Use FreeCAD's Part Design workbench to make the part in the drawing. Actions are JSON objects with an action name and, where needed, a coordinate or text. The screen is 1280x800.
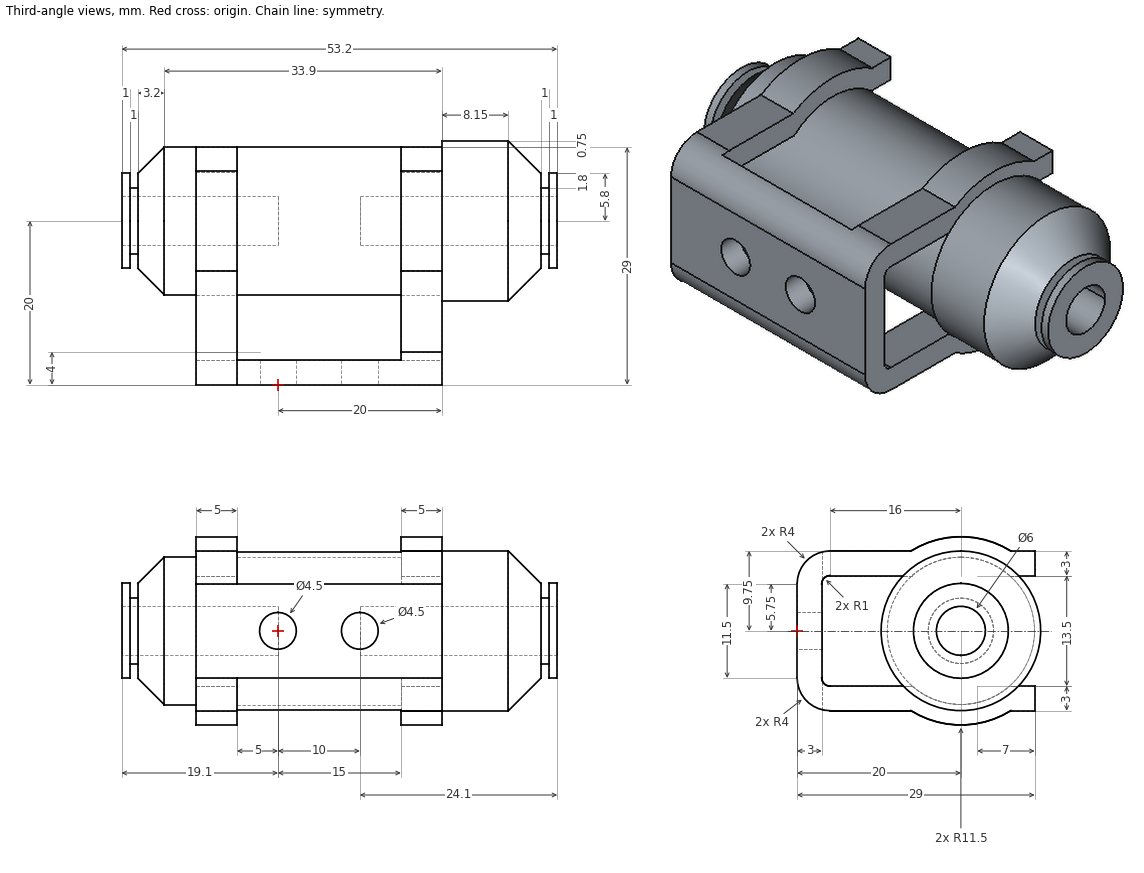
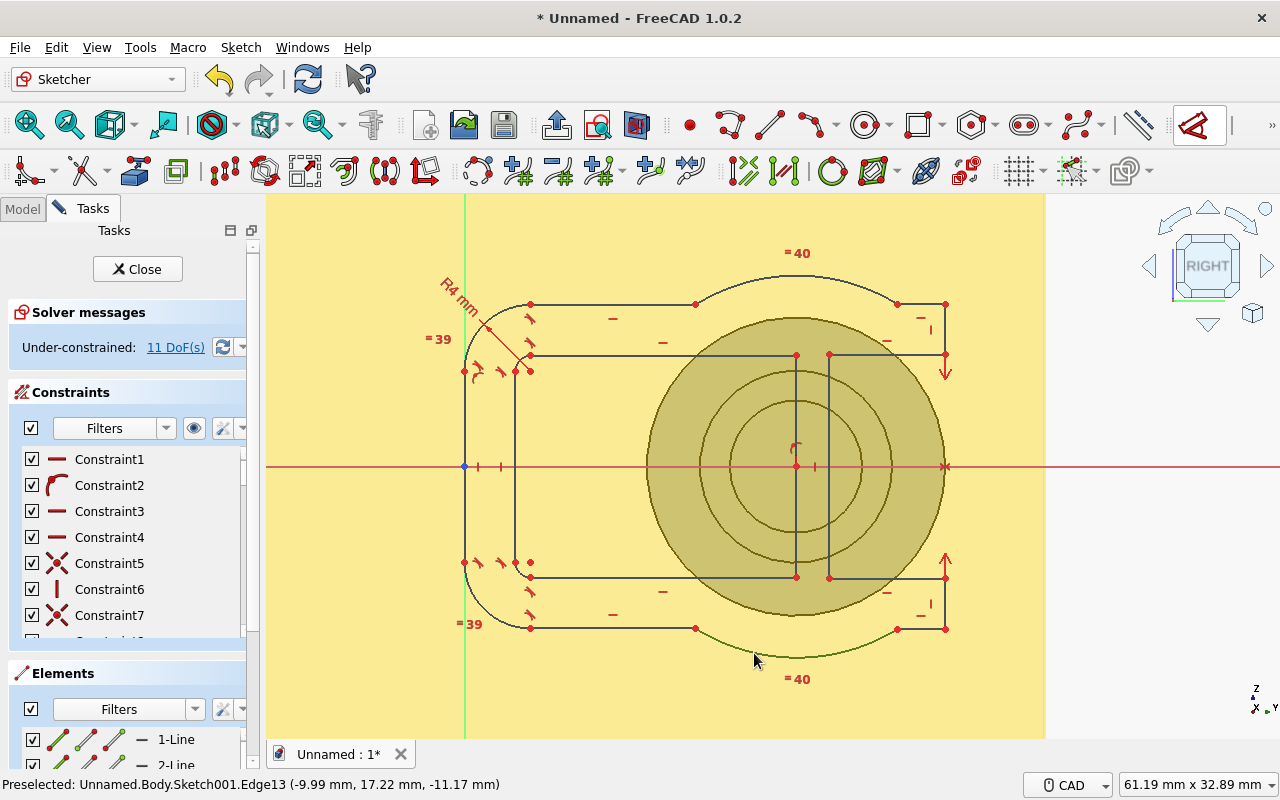
{"action": "left_click", "coordinate": [1220, 126]}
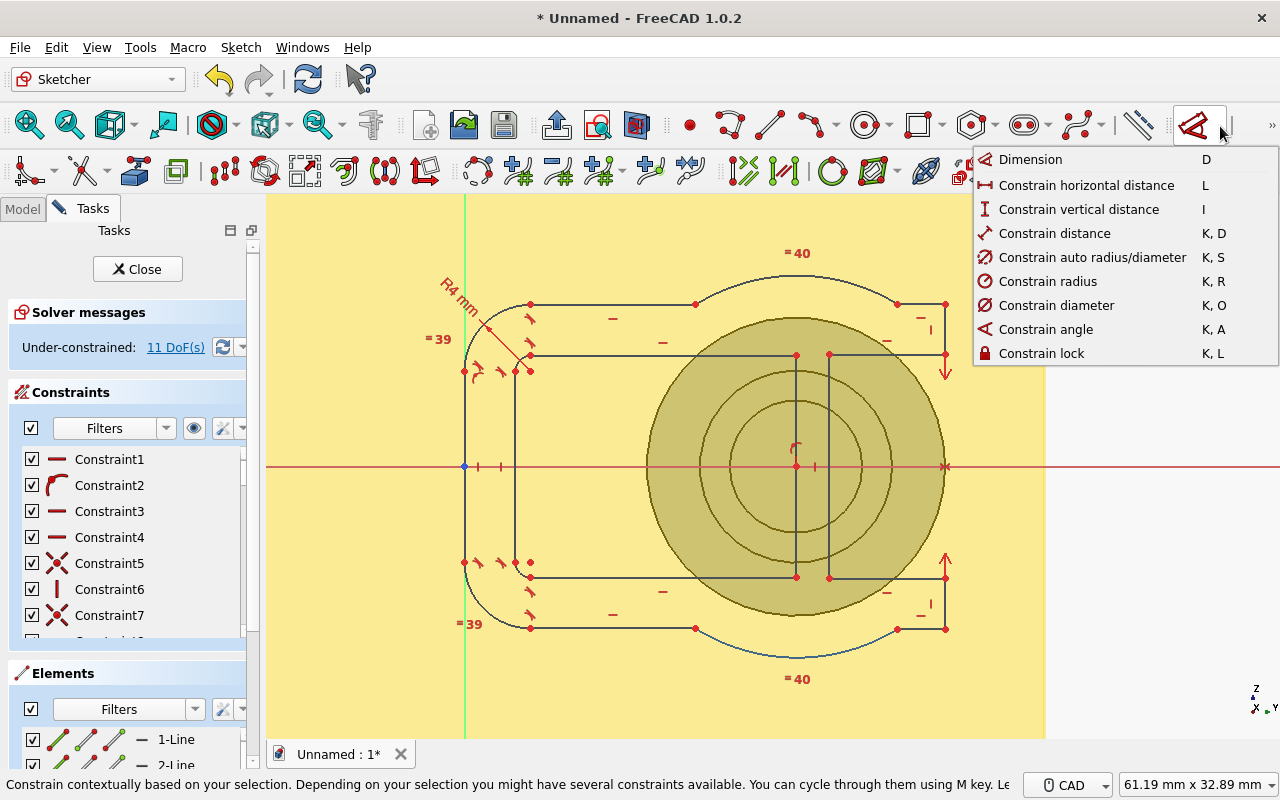
{"action": "left_click", "coordinate": [1126, 281]}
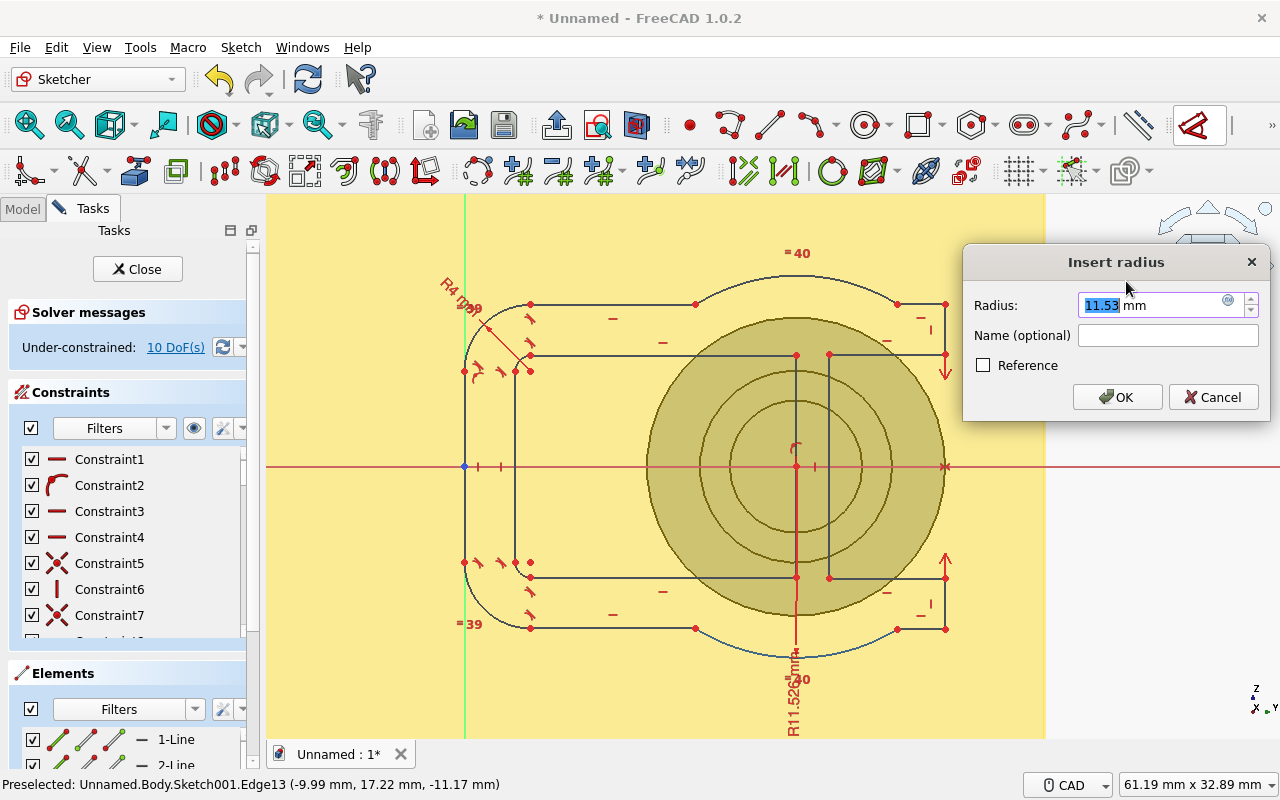
{"action": "type", "text": "11.5"}
{"action": "key", "text": "Return"}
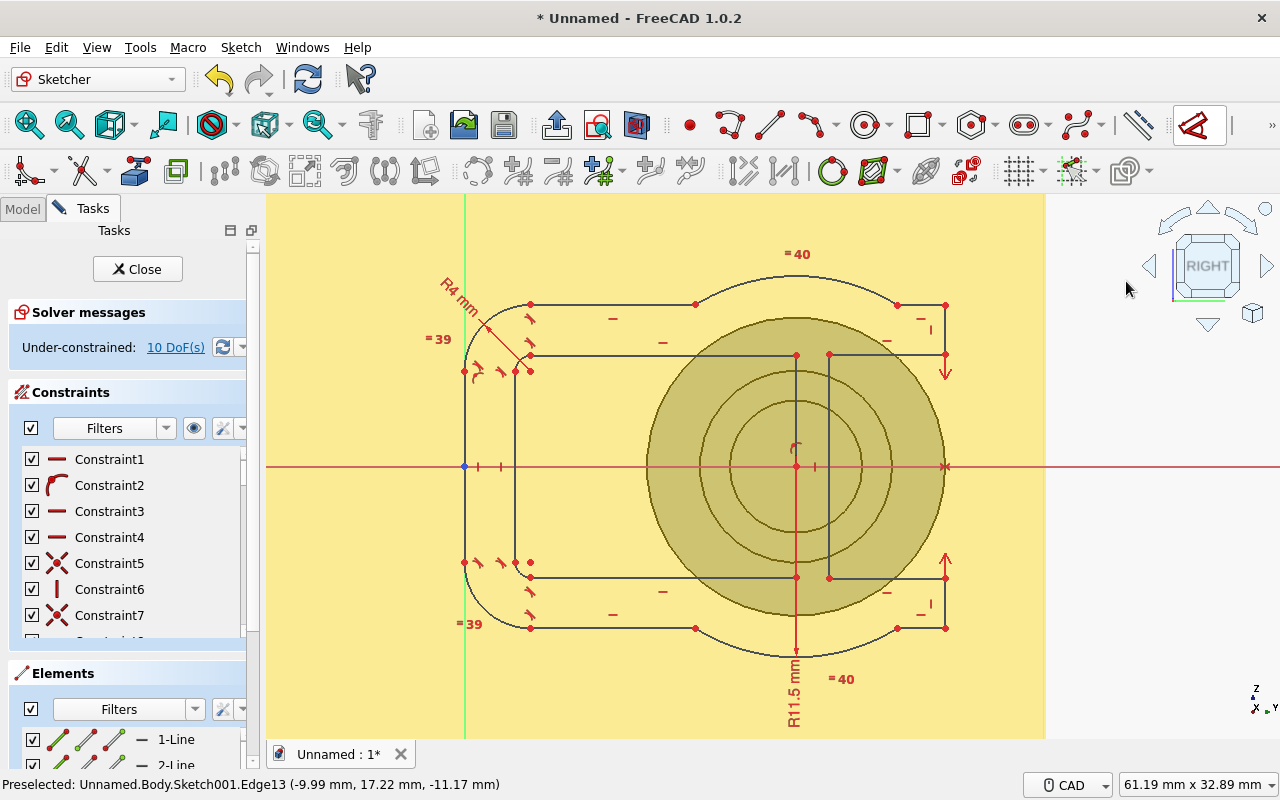
{"action": "scroll", "coordinate": [520, 360], "scroll_direction": "up", "scroll_amount": 5}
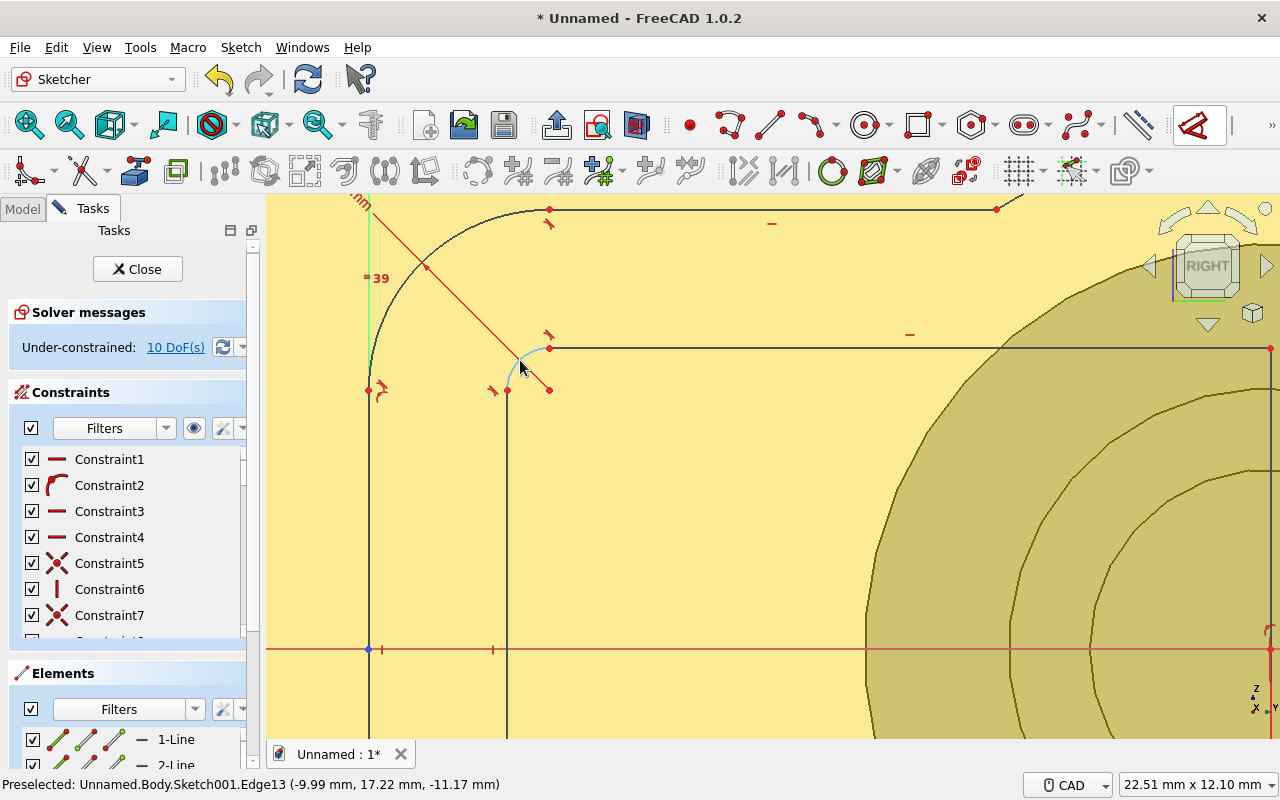
{"action": "left_click", "coordinate": [519, 360]}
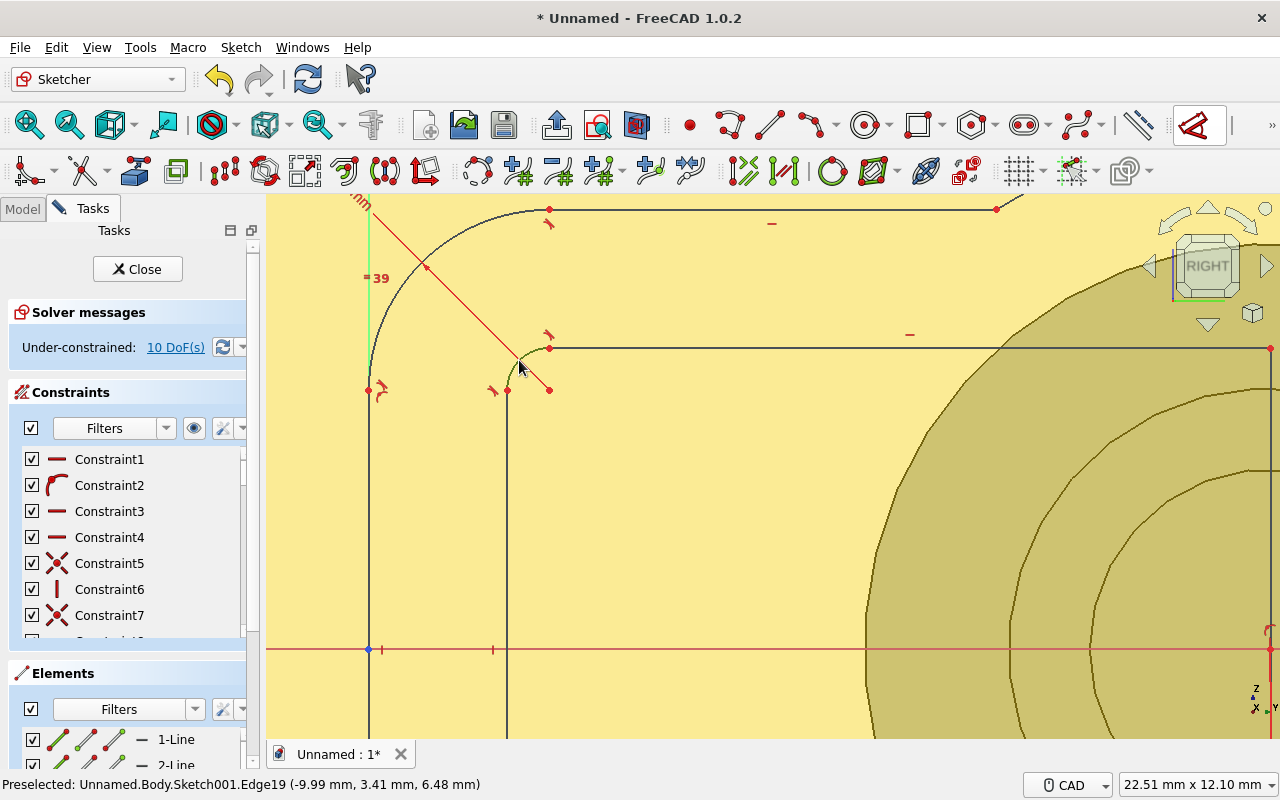
{"action": "key", "text": "k r"}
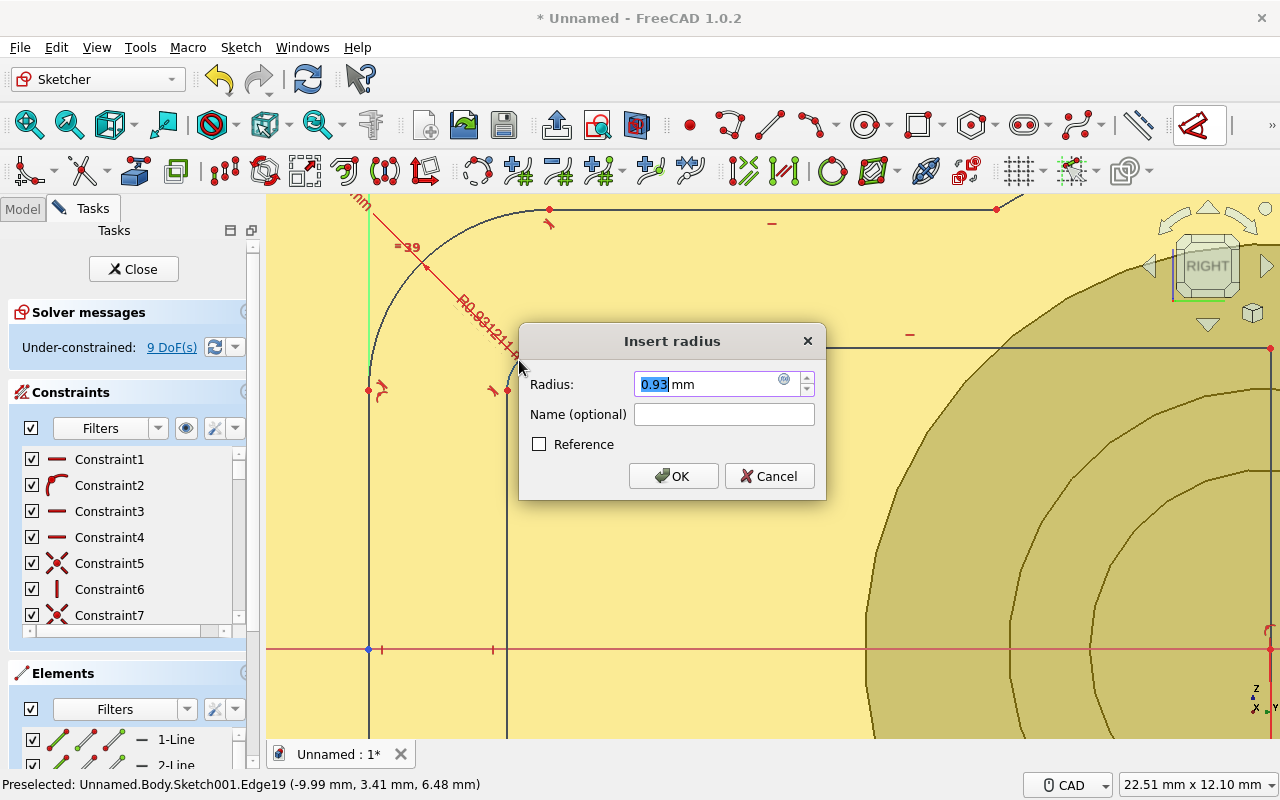
{"action": "type", "text": "1"}
{"action": "key", "text": "Return"}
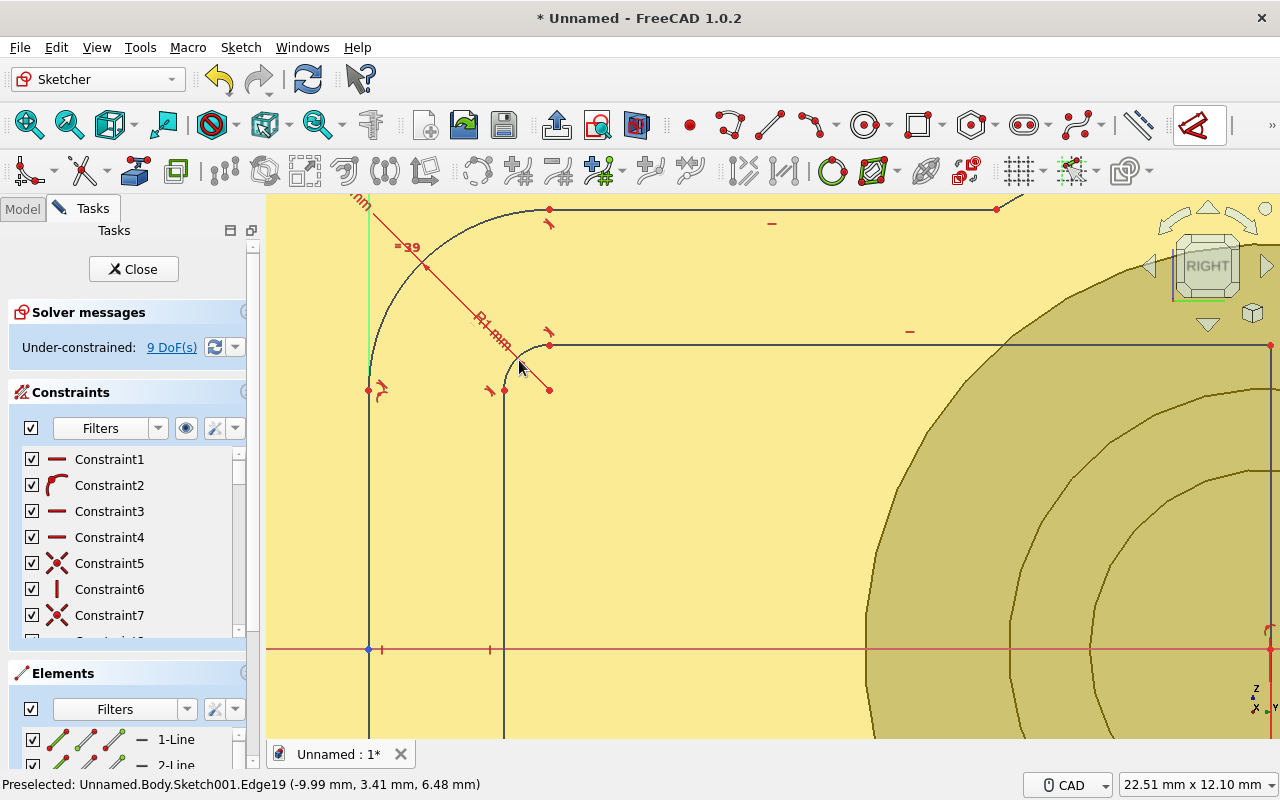
{"action": "scroll", "coordinate": [520, 360], "scroll_direction": "down", "scroll_amount": 5}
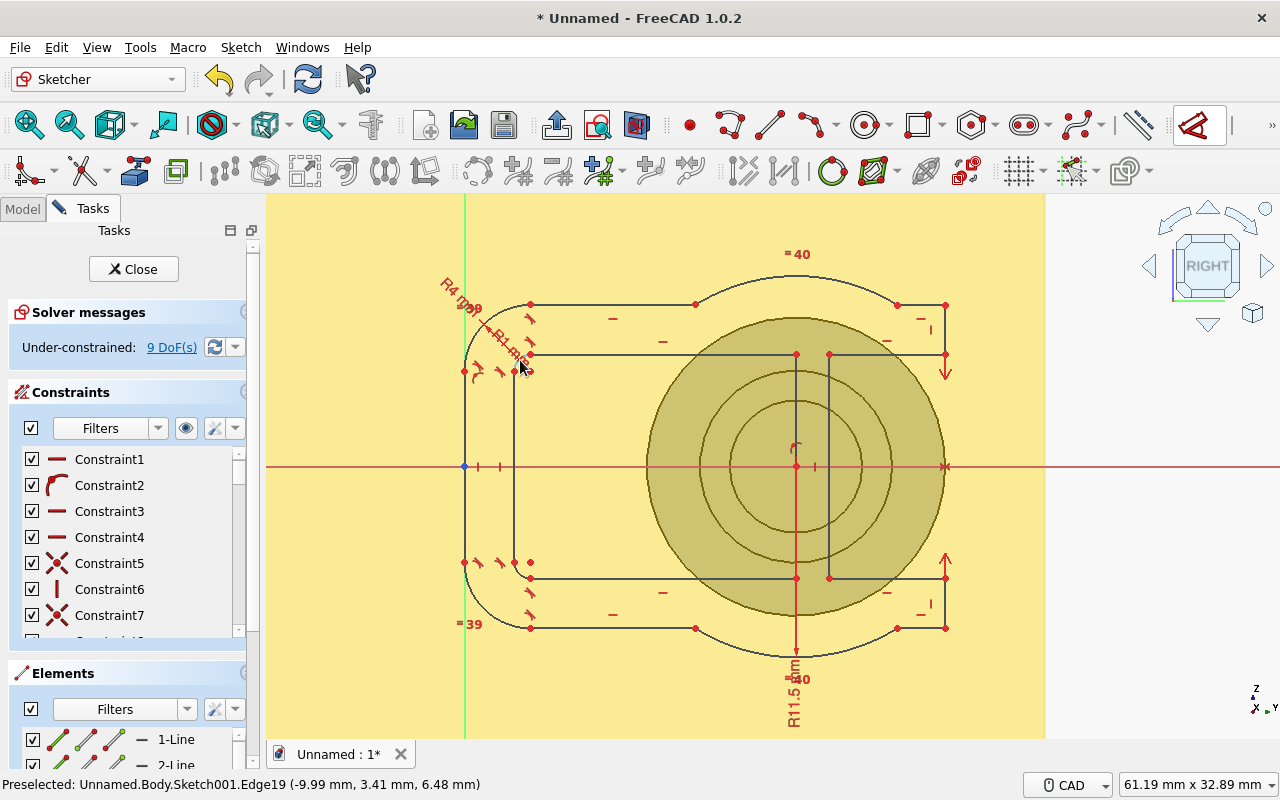
{"action": "left_click", "coordinate": [945, 613]}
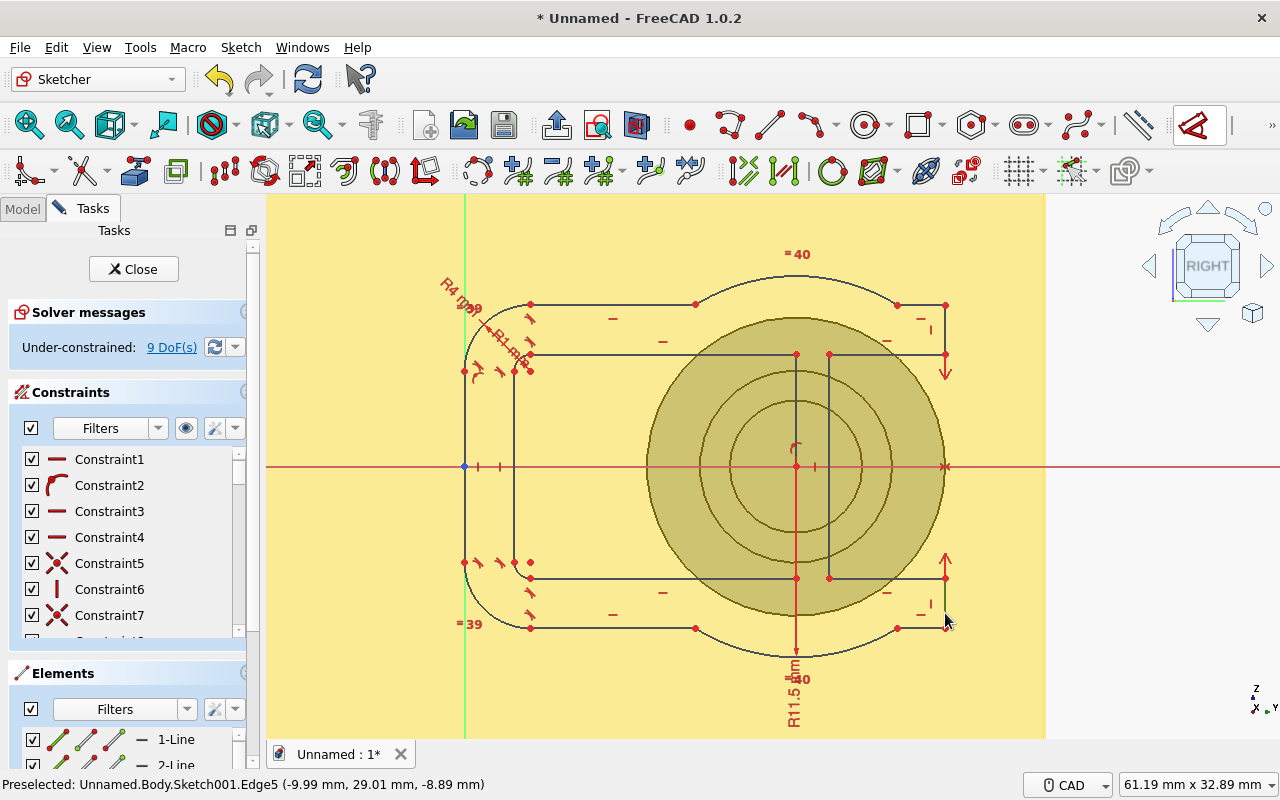
{"action": "left_click", "coordinate": [1220, 126]}